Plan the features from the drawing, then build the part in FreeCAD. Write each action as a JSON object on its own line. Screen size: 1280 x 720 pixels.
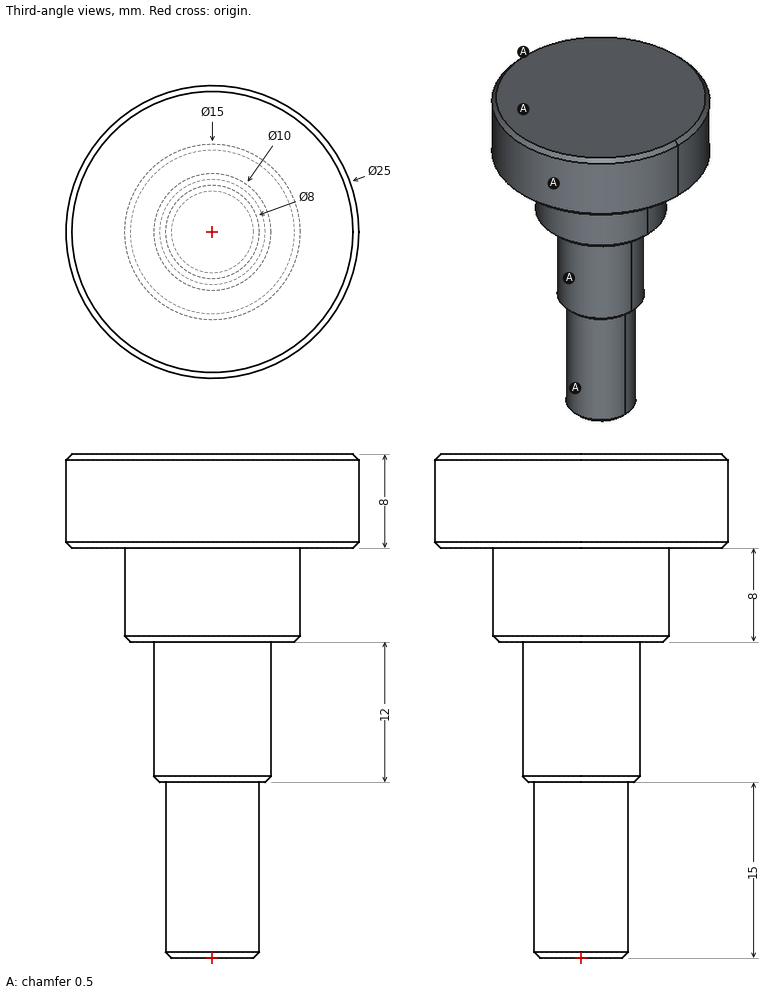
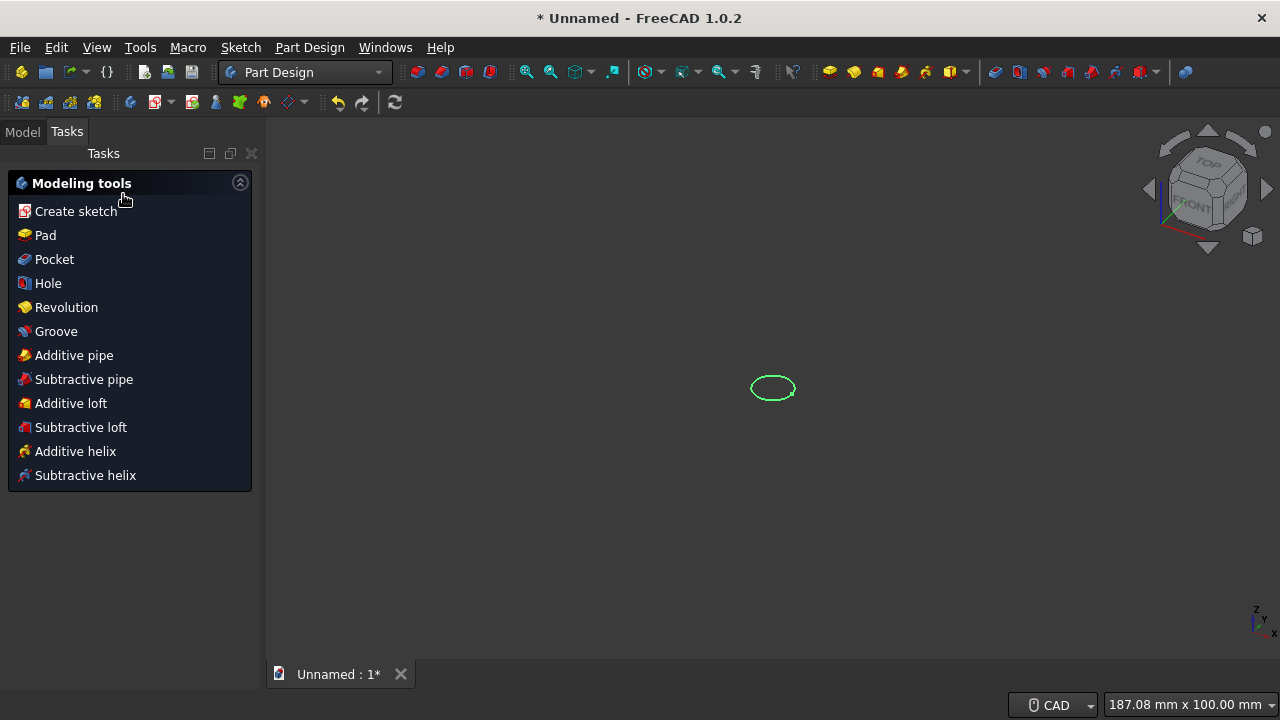
{"action": "left_click", "coordinate": [830, 72]}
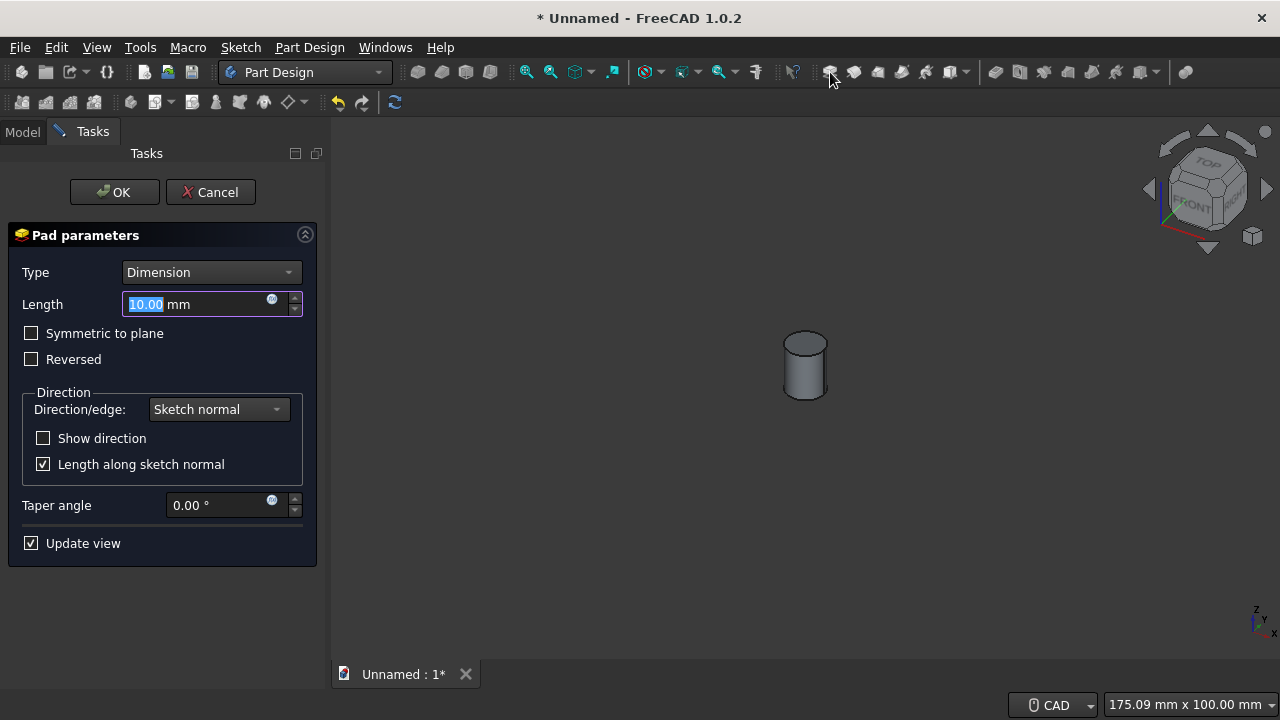
{"action": "type", "text": "15"}
{"action": "key", "text": "Tab"}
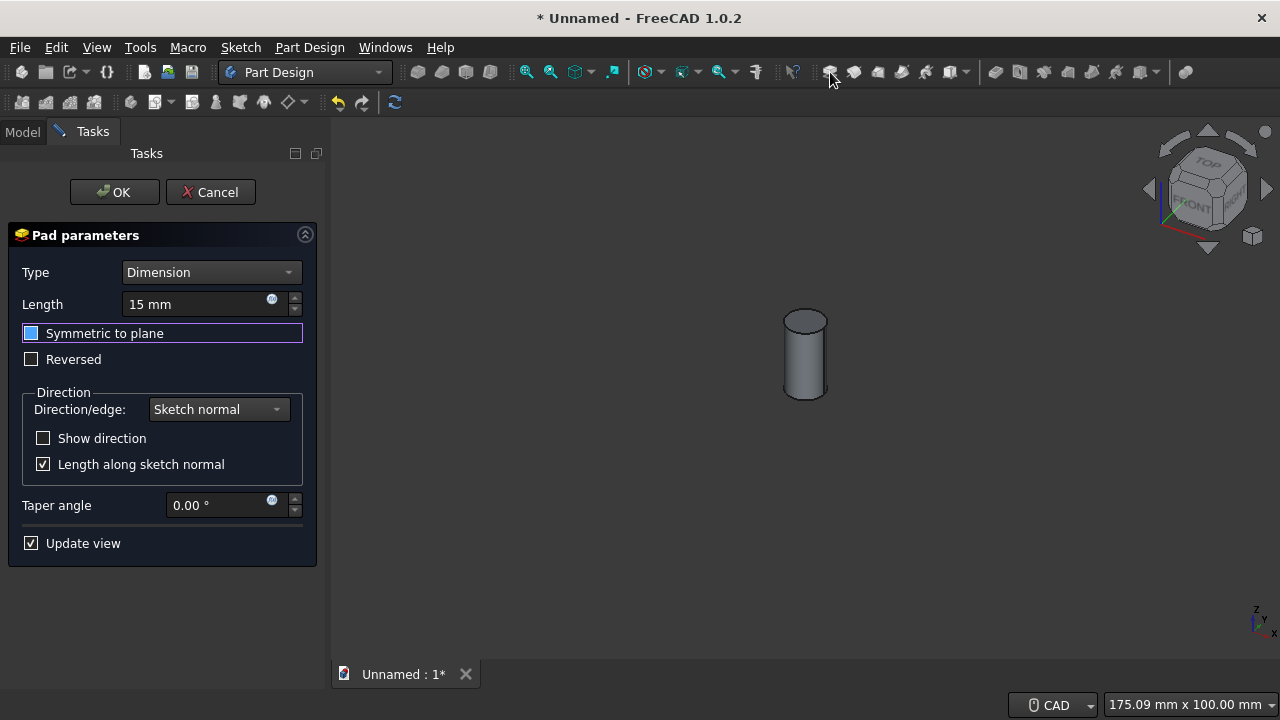
{"action": "left_click", "coordinate": [115, 192]}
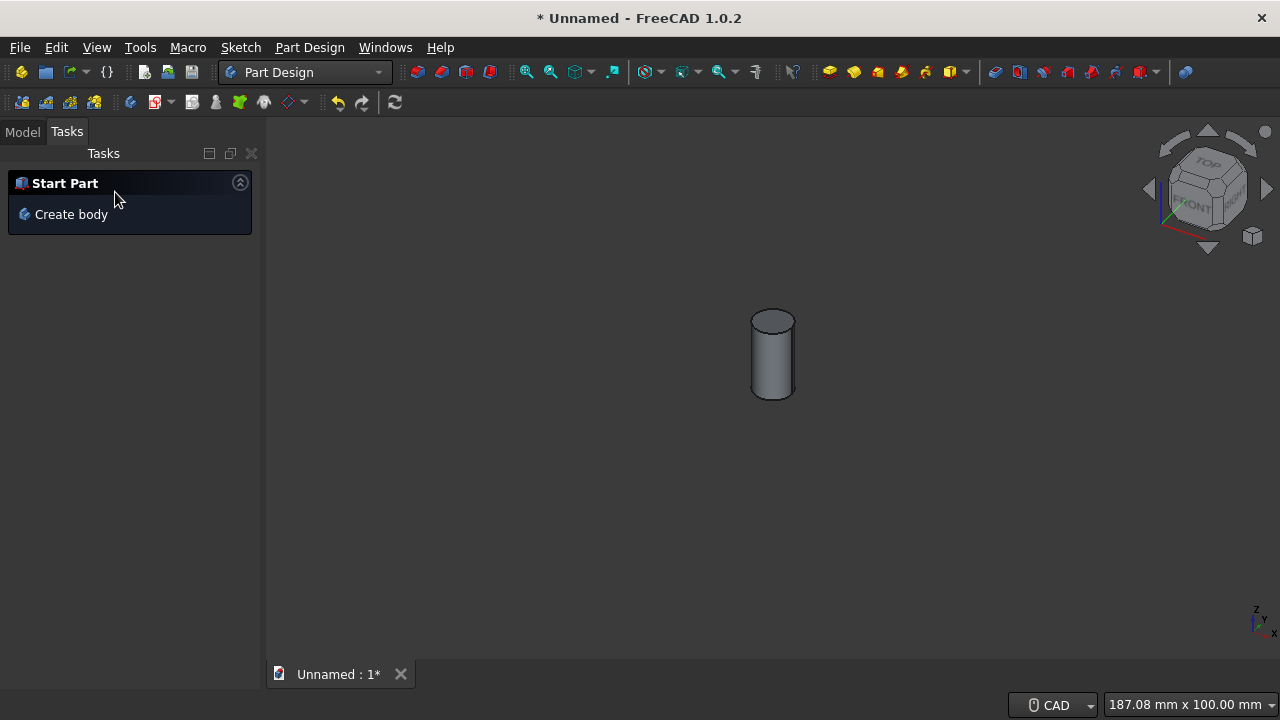
{"action": "left_click", "coordinate": [528, 72]}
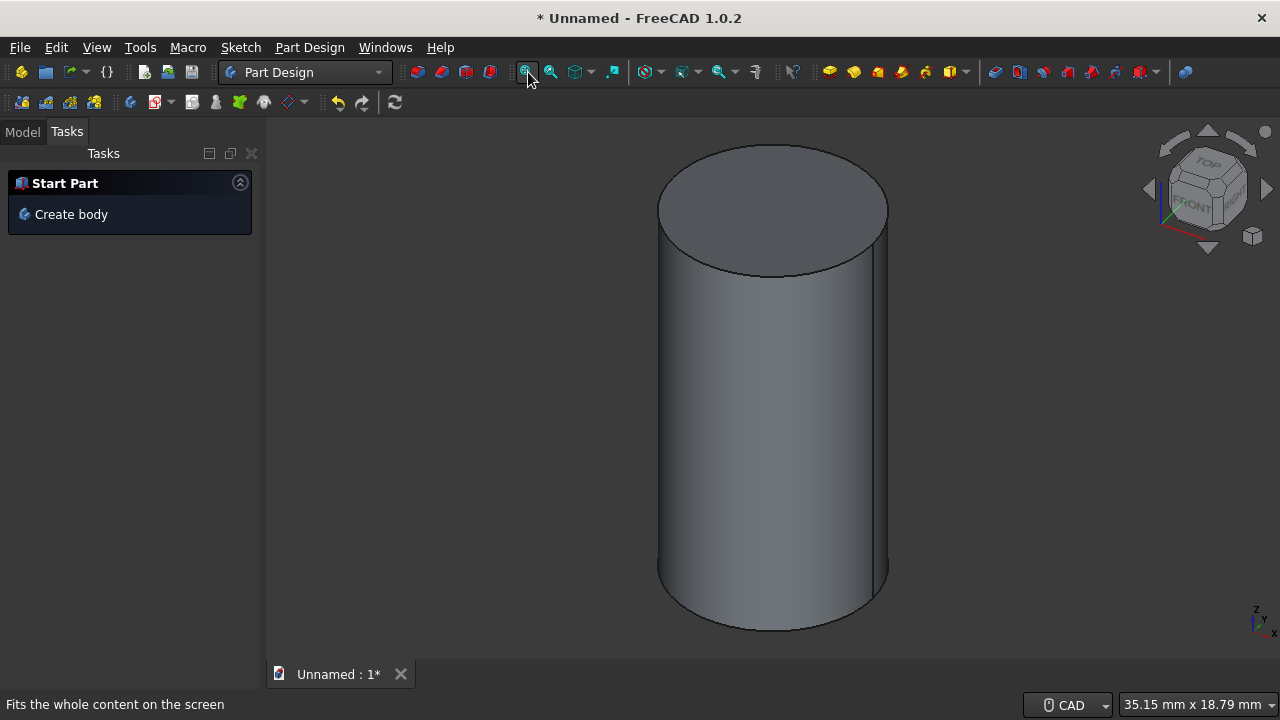
{"action": "left_click", "coordinate": [773, 210]}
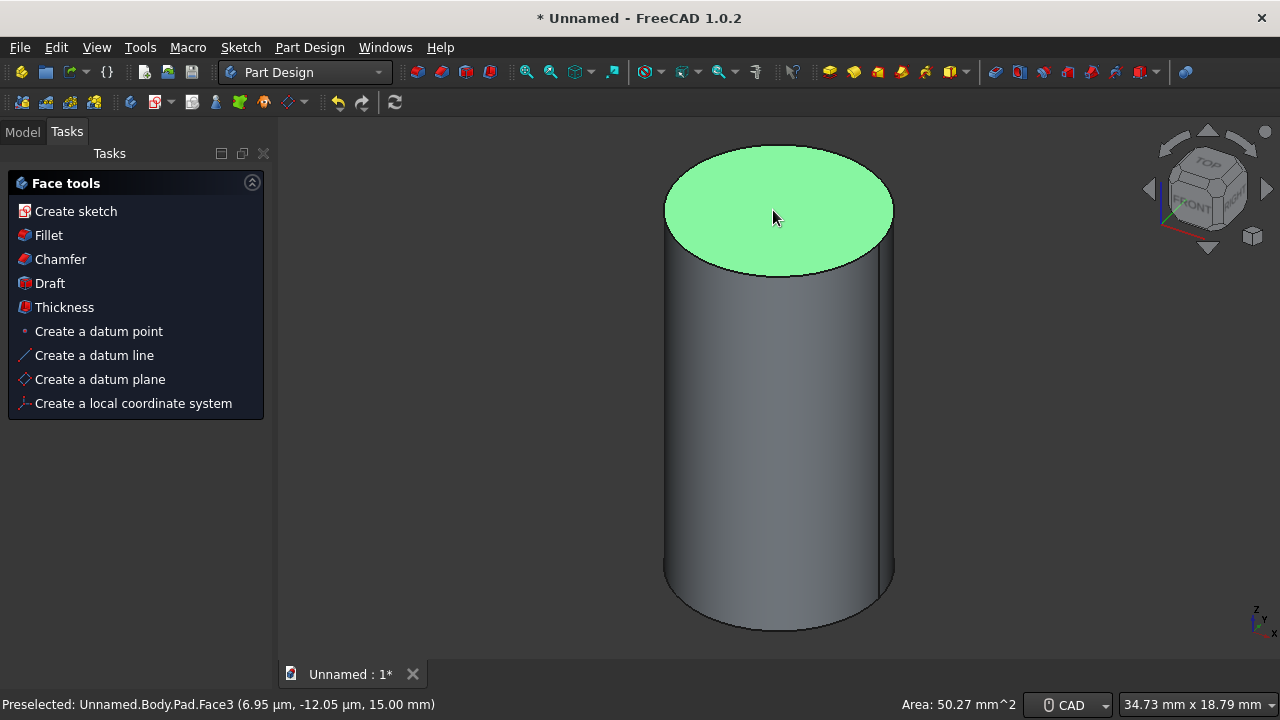
{"action": "left_click", "coordinate": [156, 102]}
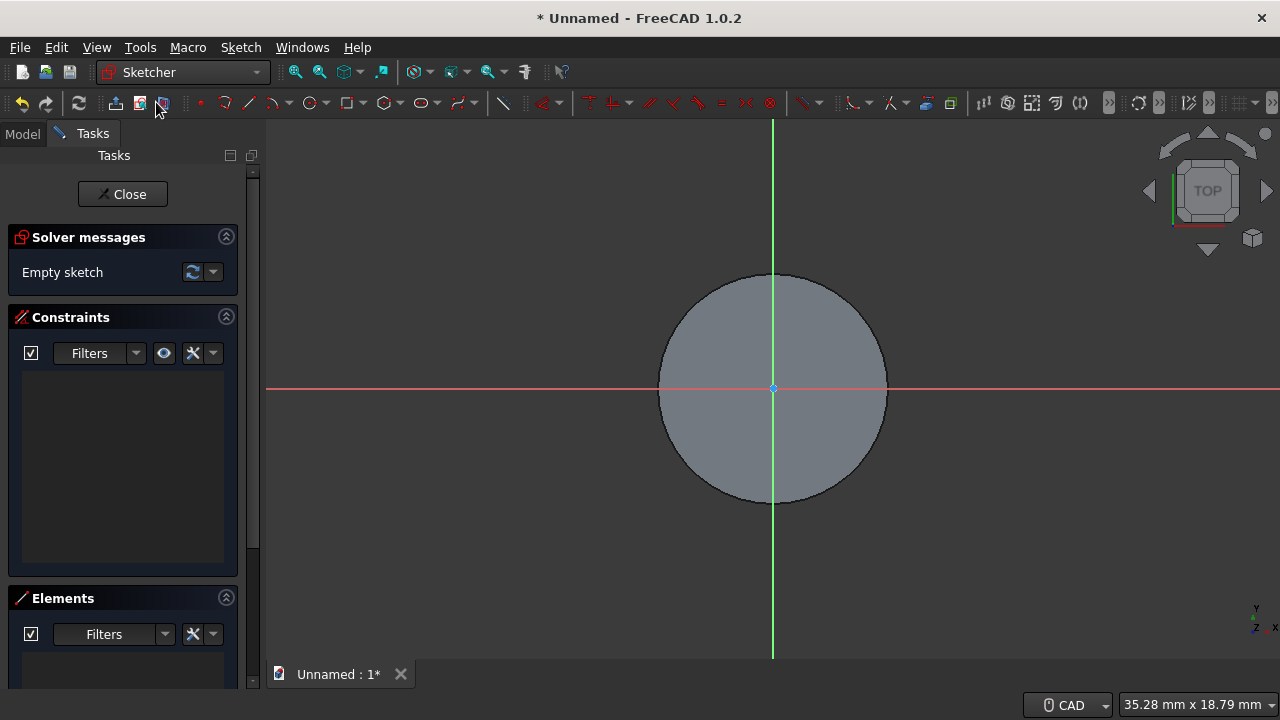
{"action": "left_click", "coordinate": [310, 104]}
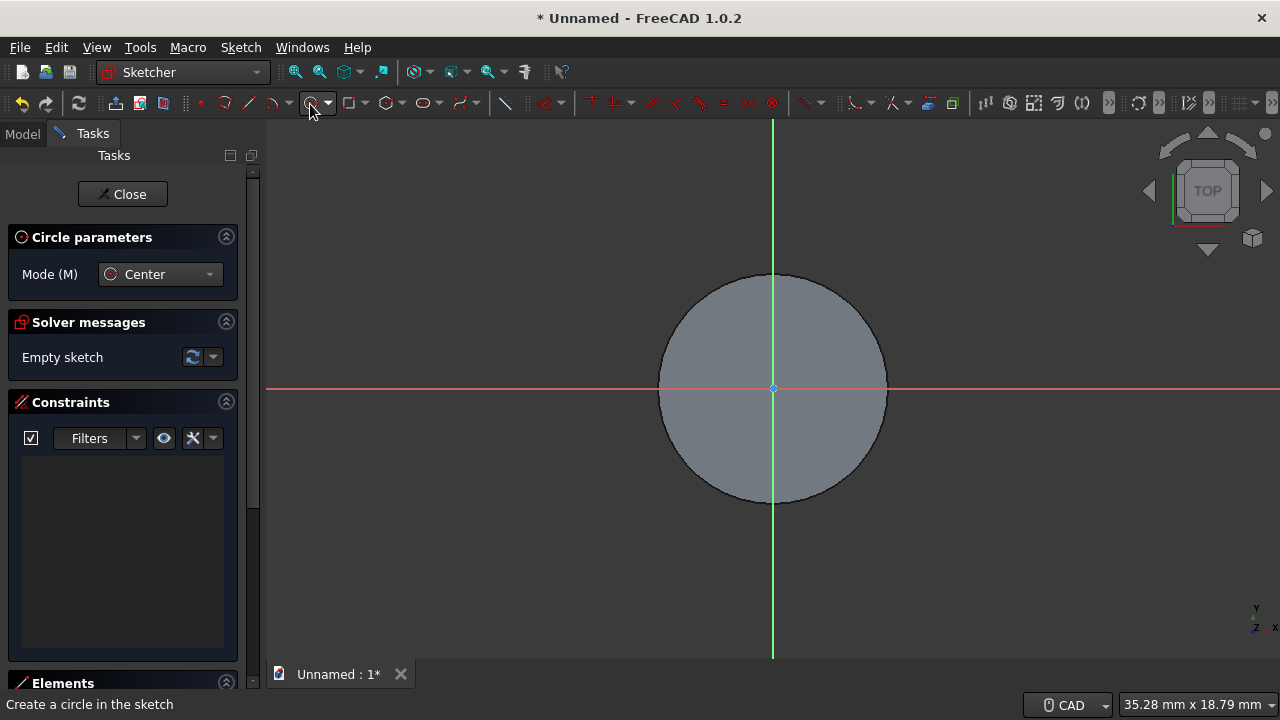
{"action": "left_click", "coordinate": [773, 389]}
{"action": "left_click", "coordinate": [875, 287]}
{"action": "key", "text": "Escape"}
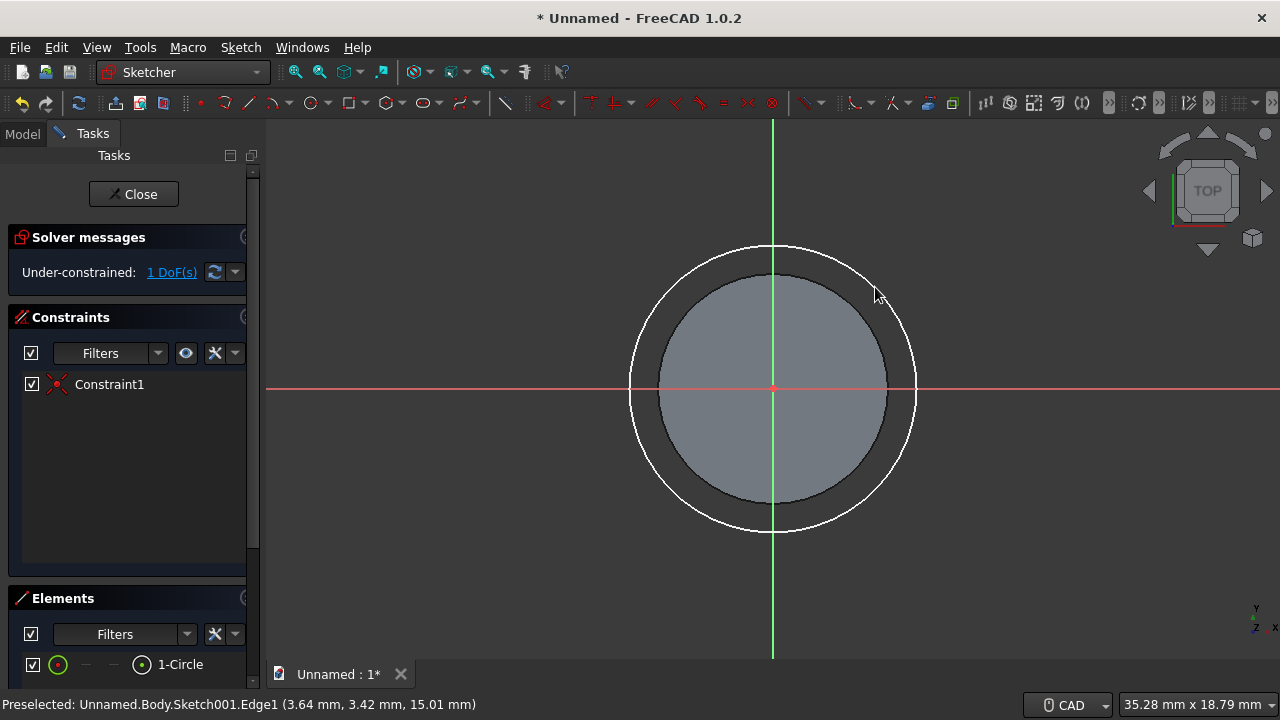
{"action": "key", "text": "d"}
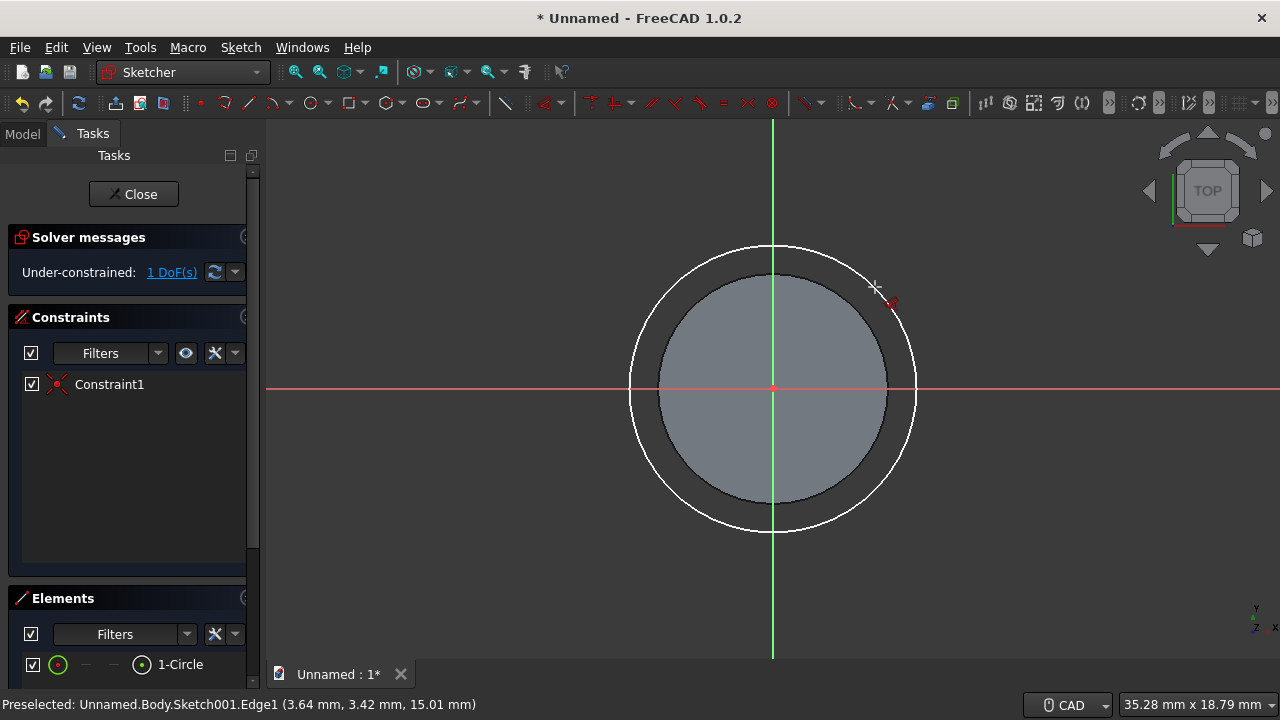
{"action": "left_click", "coordinate": [874, 287]}
{"action": "left_click", "coordinate": [897, 264]}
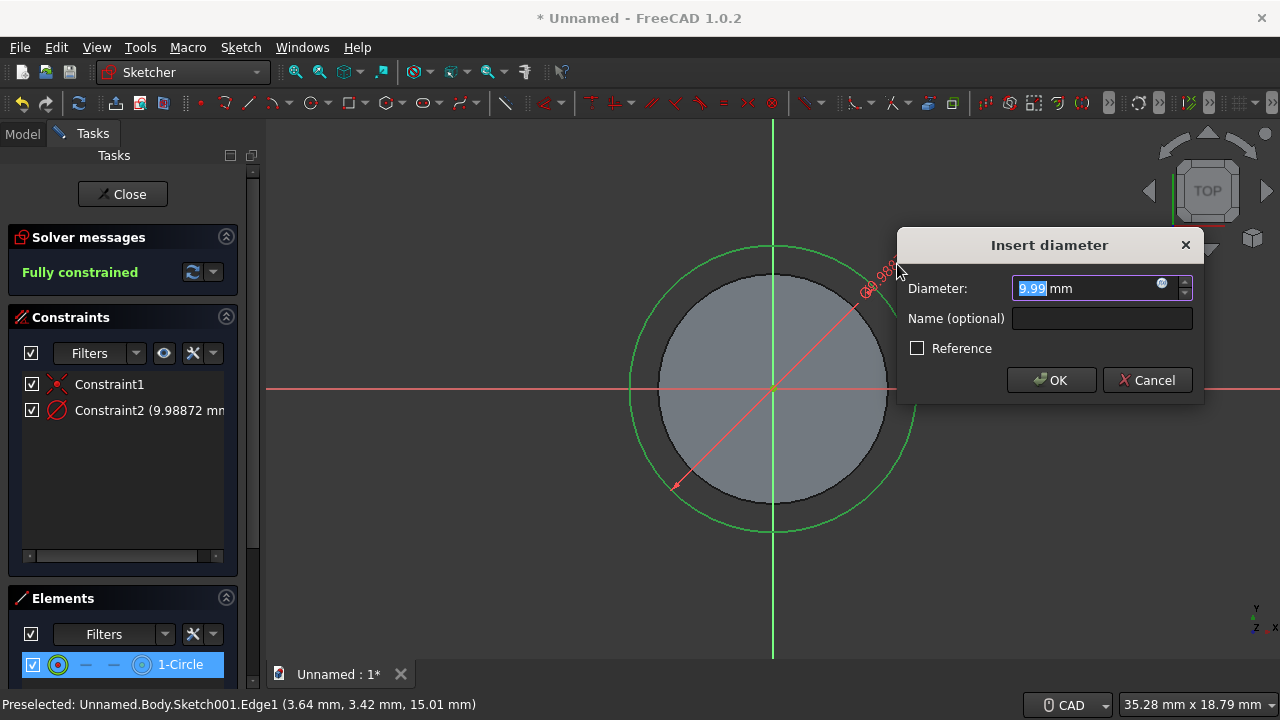
{"action": "type", "text": "10"}
{"action": "key", "text": "Return"}
{"action": "key", "text": "Escape"}